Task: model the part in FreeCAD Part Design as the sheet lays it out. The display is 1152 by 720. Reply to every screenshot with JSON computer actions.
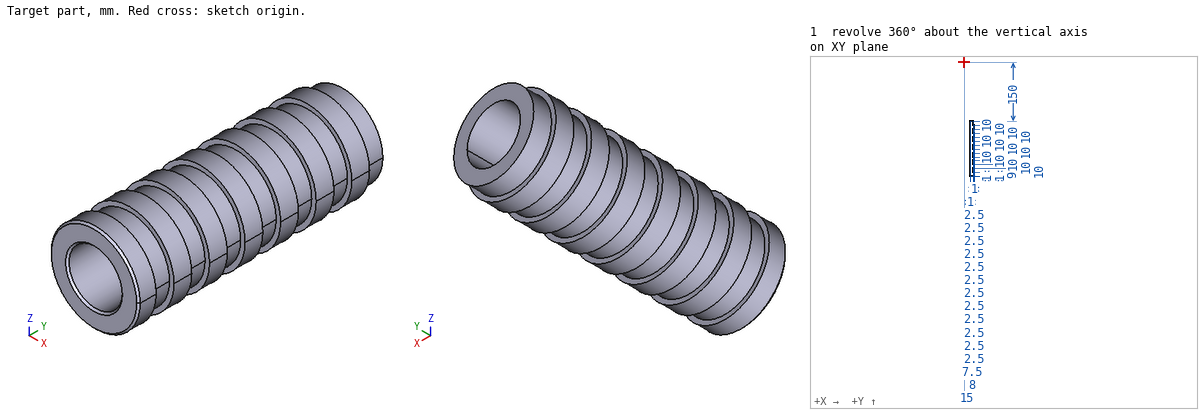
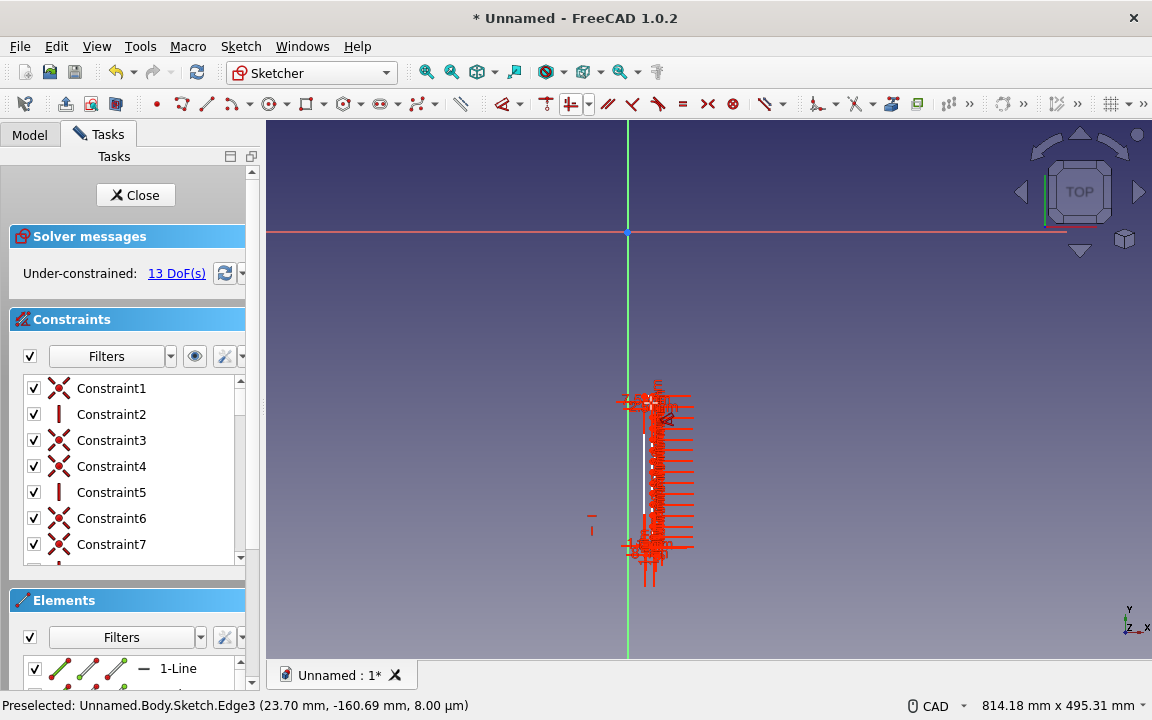
{"action": "scroll", "coordinate": [654, 418], "scroll_direction": "up", "scroll_amount": 14}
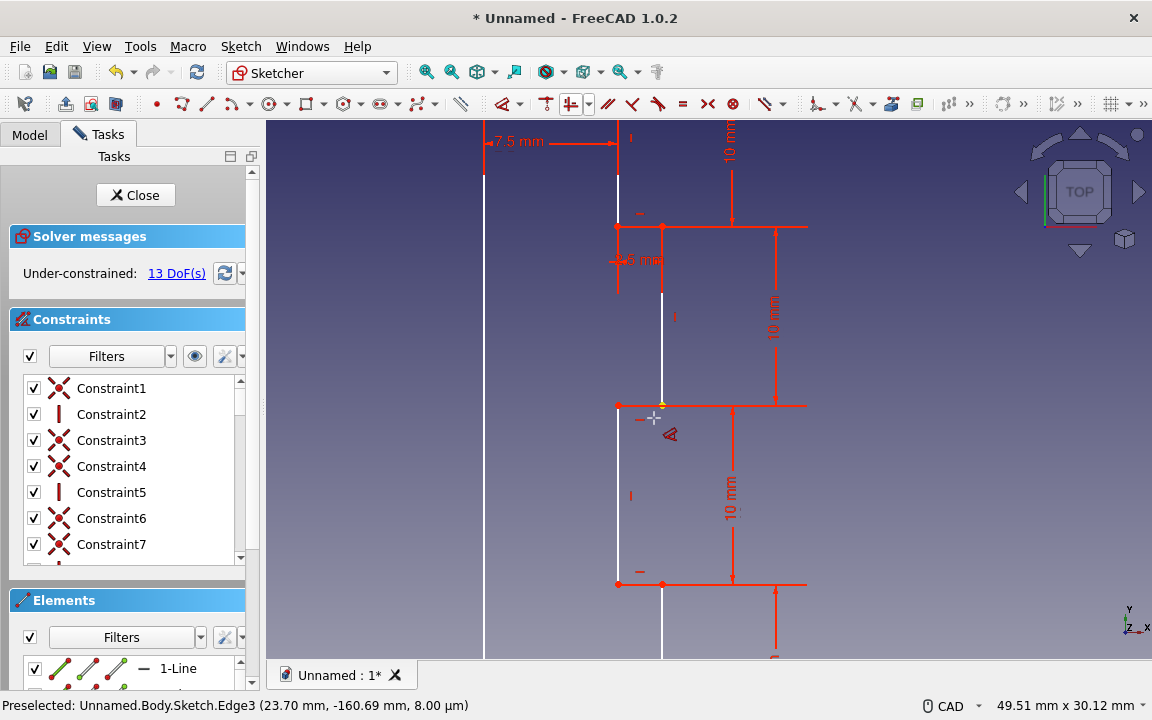
{"action": "left_click", "coordinate": [649, 406]}
{"action": "left_click", "coordinate": [640, 440]}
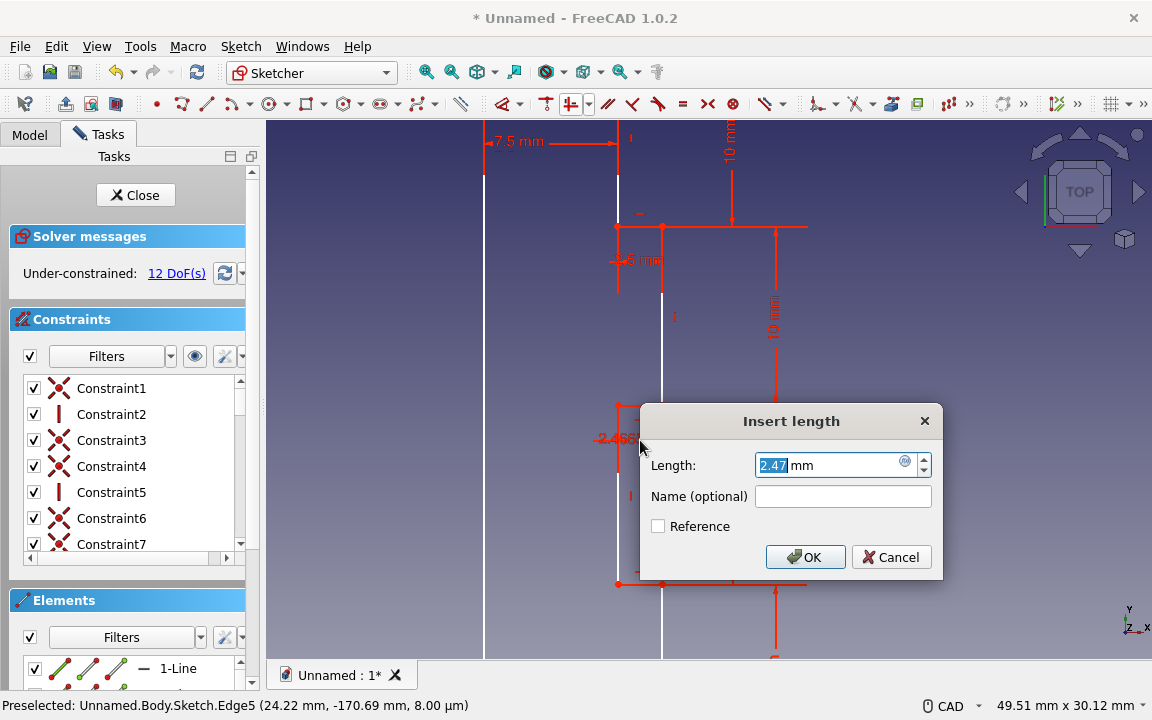
{"action": "type", "text": "2.5"}
{"action": "key", "text": "Return"}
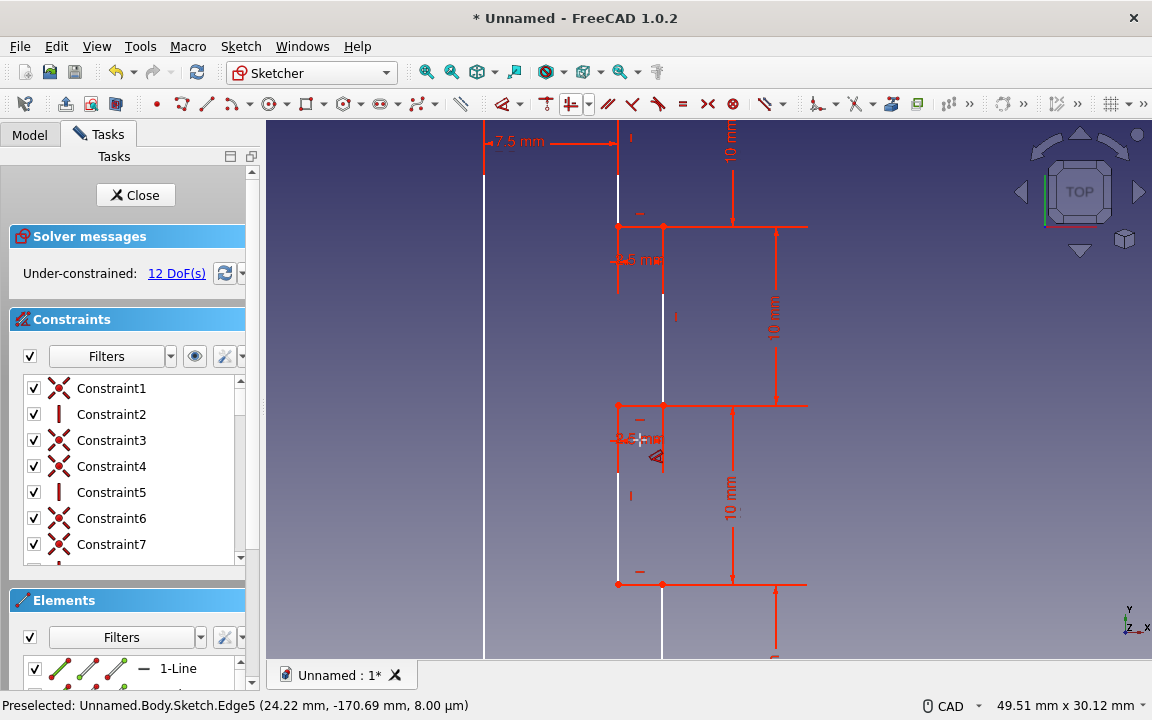
{"action": "left_click", "coordinate": [632, 585]}
{"action": "left_click", "coordinate": [640, 619]}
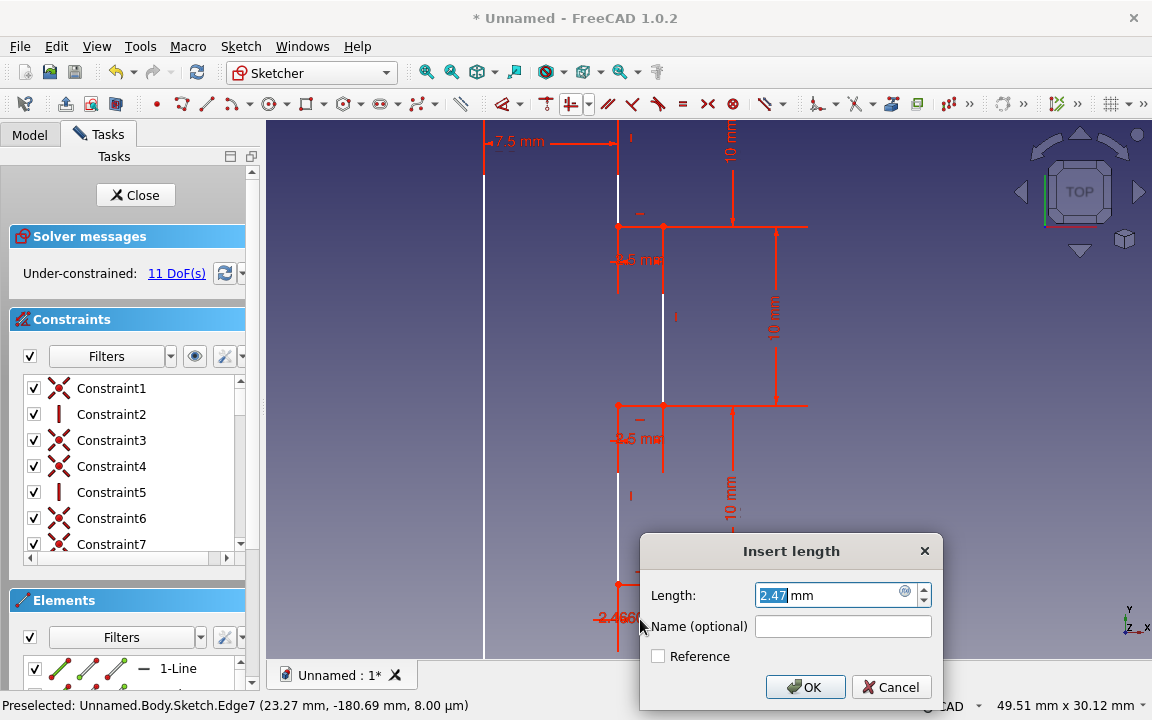
{"action": "type", "text": "2.5"}
{"action": "key", "text": "Return"}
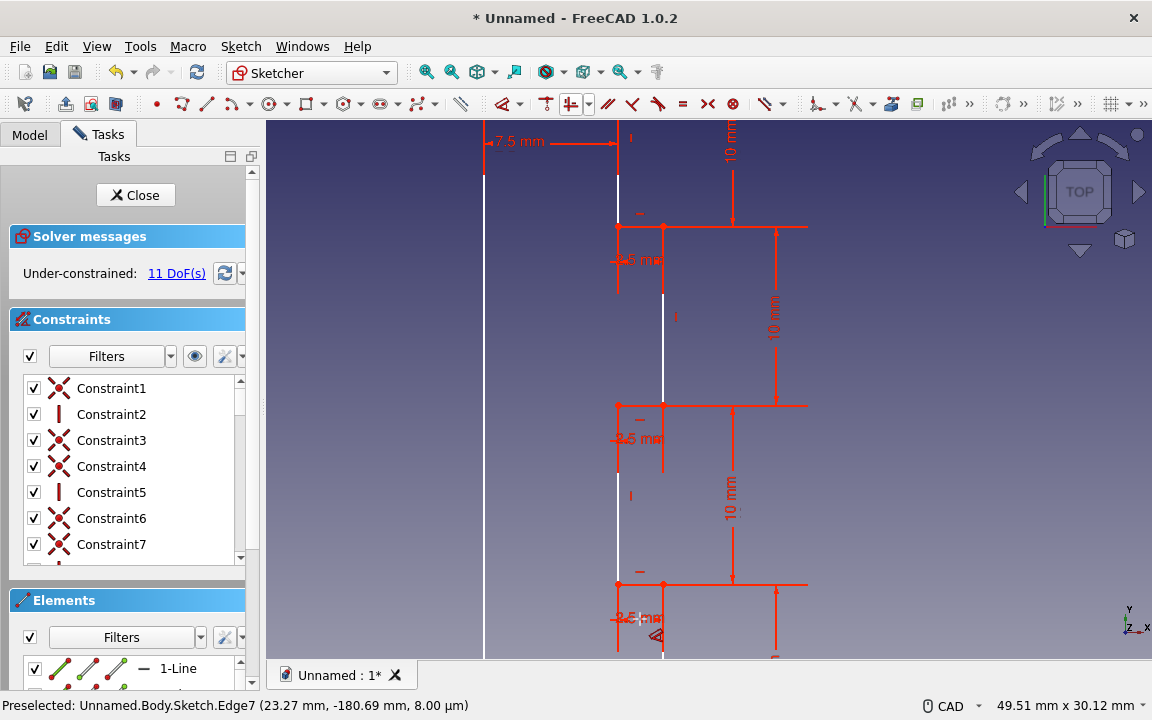
{"action": "scroll", "coordinate": [654, 418], "scroll_direction": "down", "scroll_amount": 14}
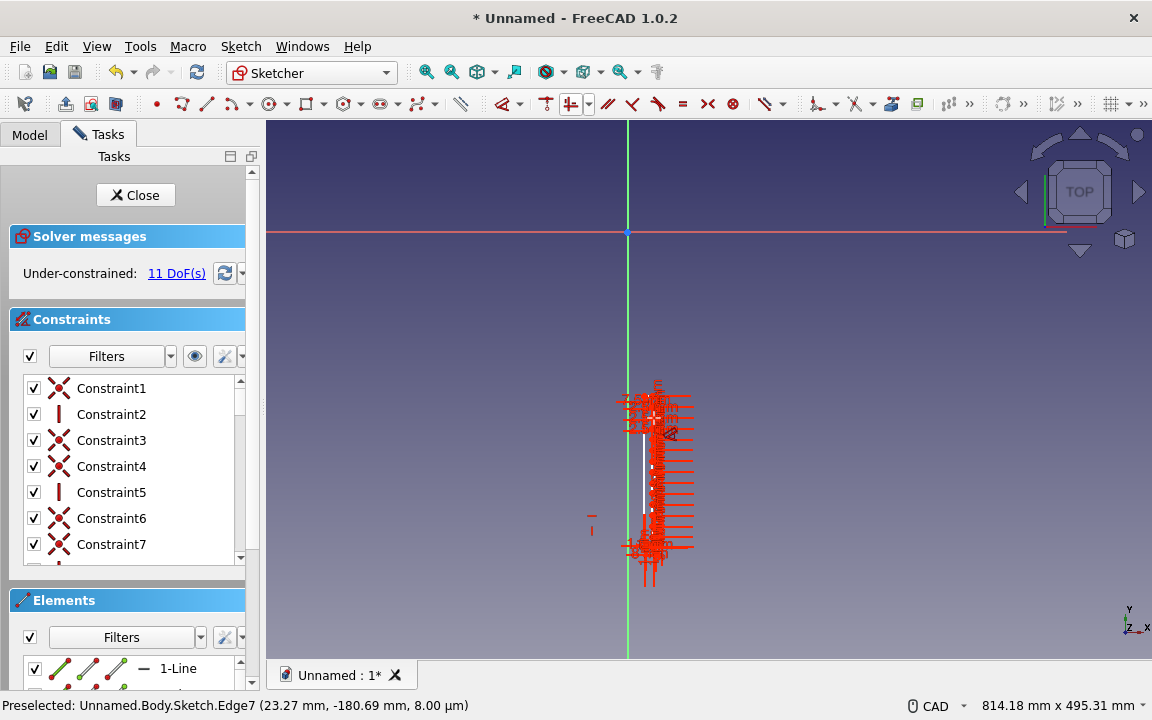
{"action": "scroll", "coordinate": [654, 440], "scroll_direction": "up", "scroll_amount": 14}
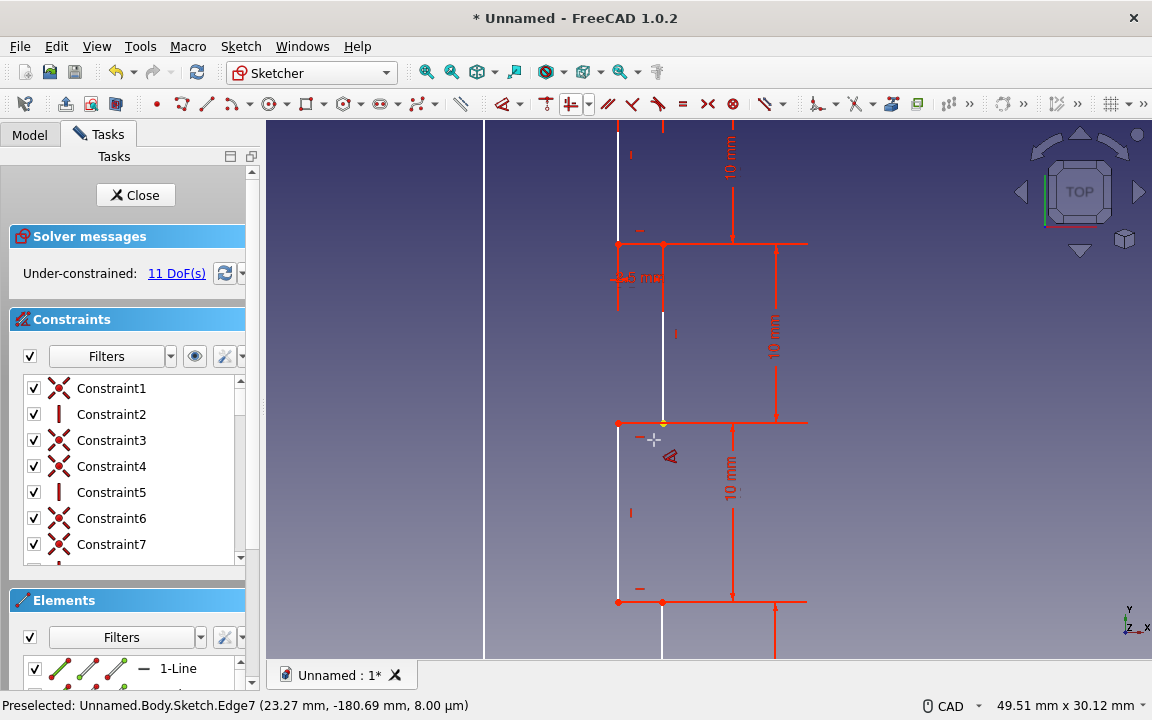
{"action": "left_click", "coordinate": [650, 423]}
{"action": "left_click", "coordinate": [641, 457]}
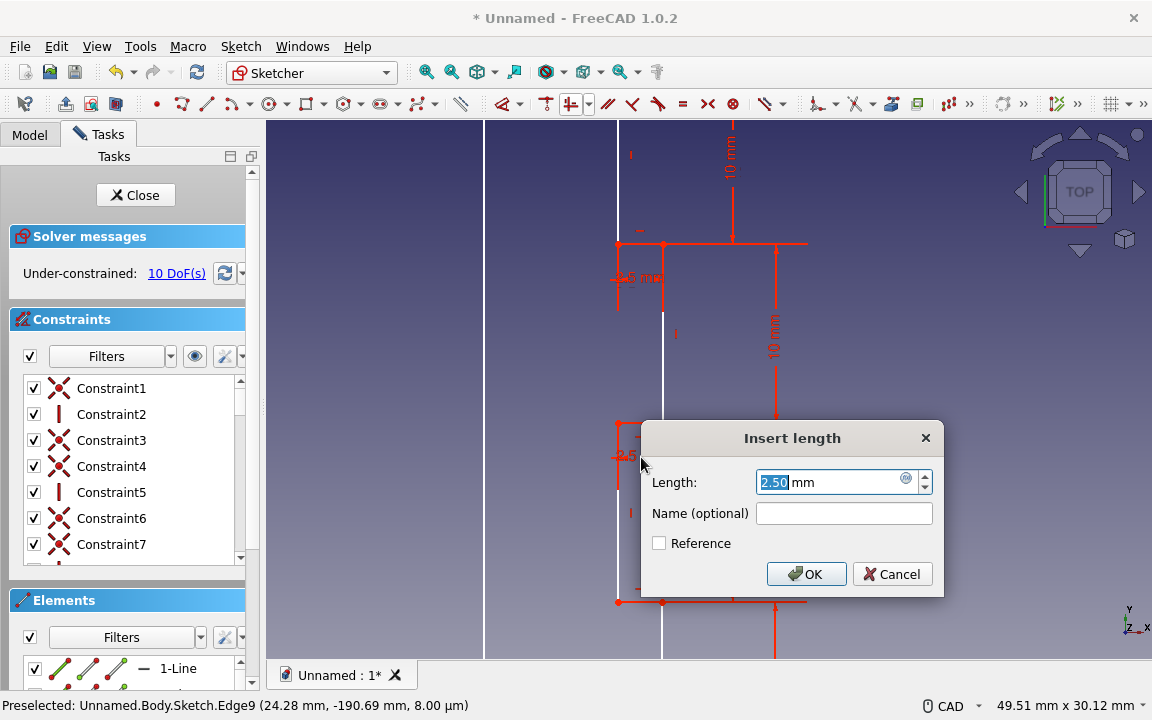
{"action": "type", "text": "2.5"}
{"action": "key", "text": "Return"}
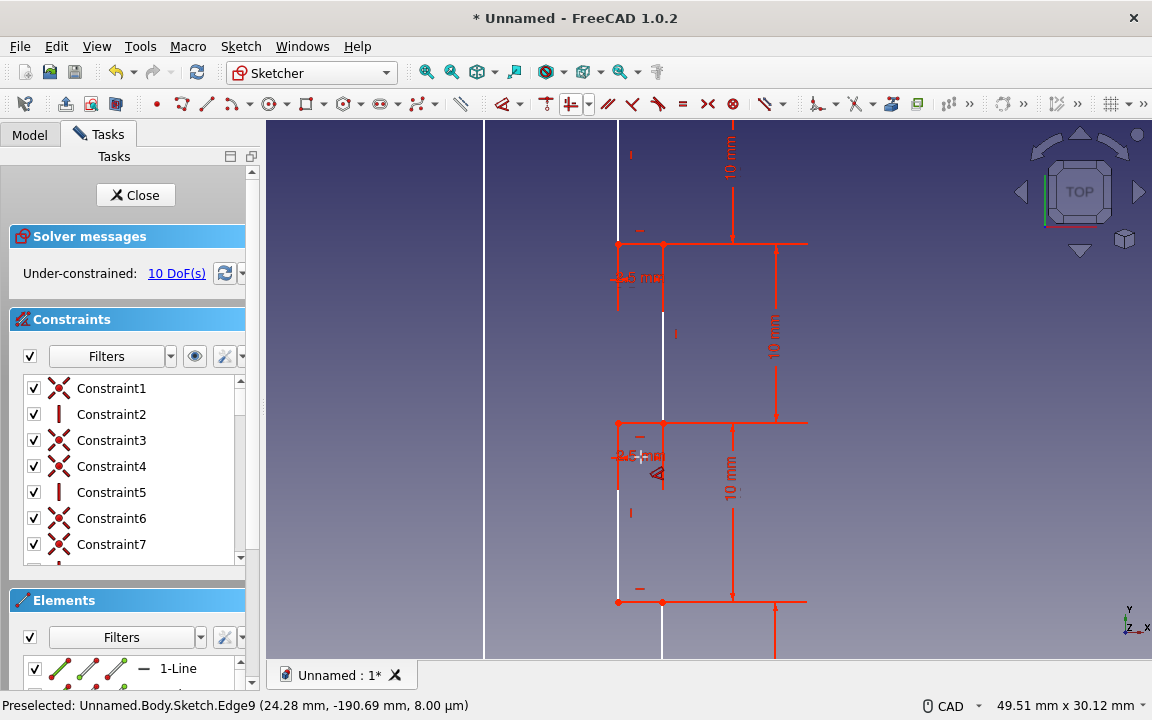
{"action": "left_click", "coordinate": [632, 602]}
{"action": "left_click", "coordinate": [640, 568]}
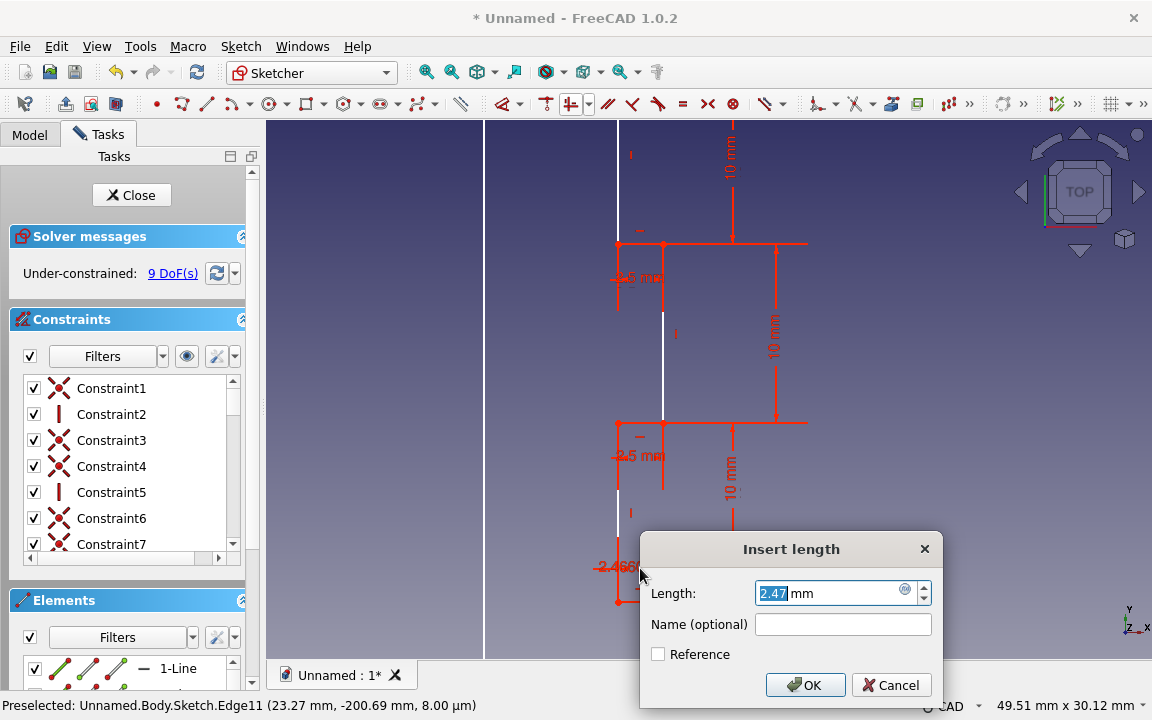
{"action": "type", "text": "2.5"}
{"action": "key", "text": "Return"}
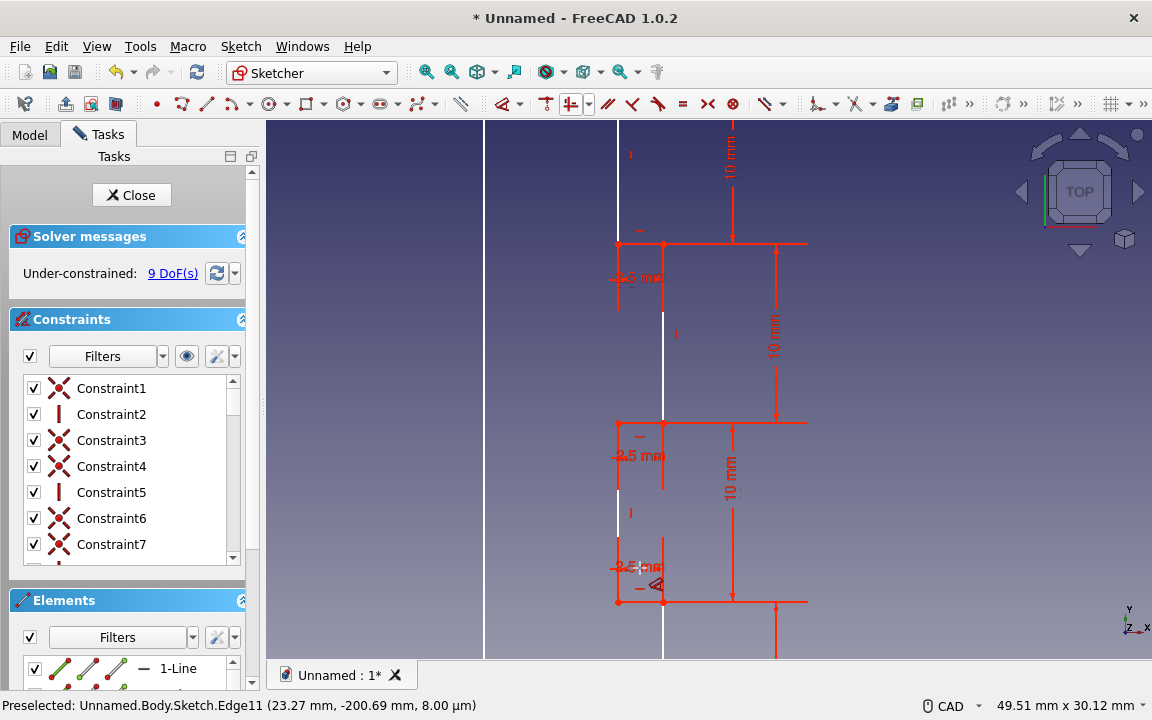
{"action": "scroll", "coordinate": [654, 440], "scroll_direction": "down", "scroll_amount": 14}